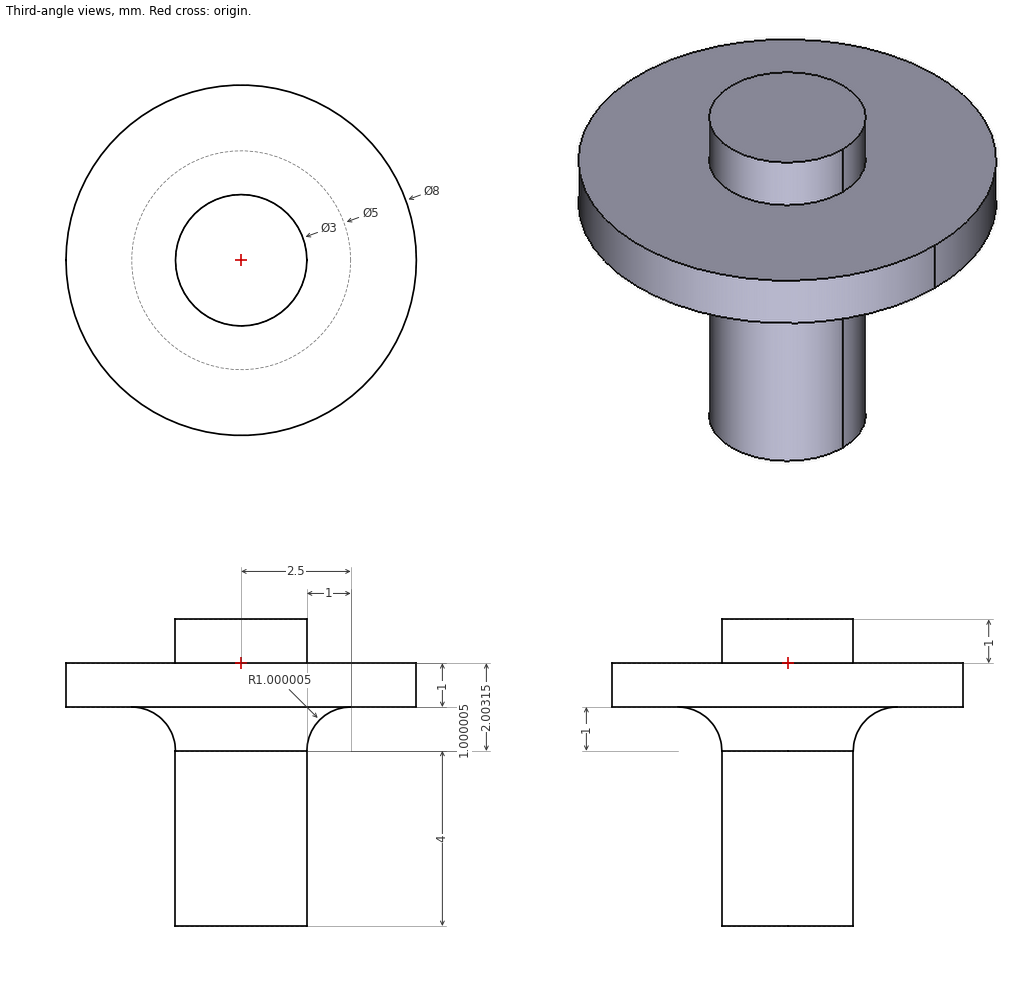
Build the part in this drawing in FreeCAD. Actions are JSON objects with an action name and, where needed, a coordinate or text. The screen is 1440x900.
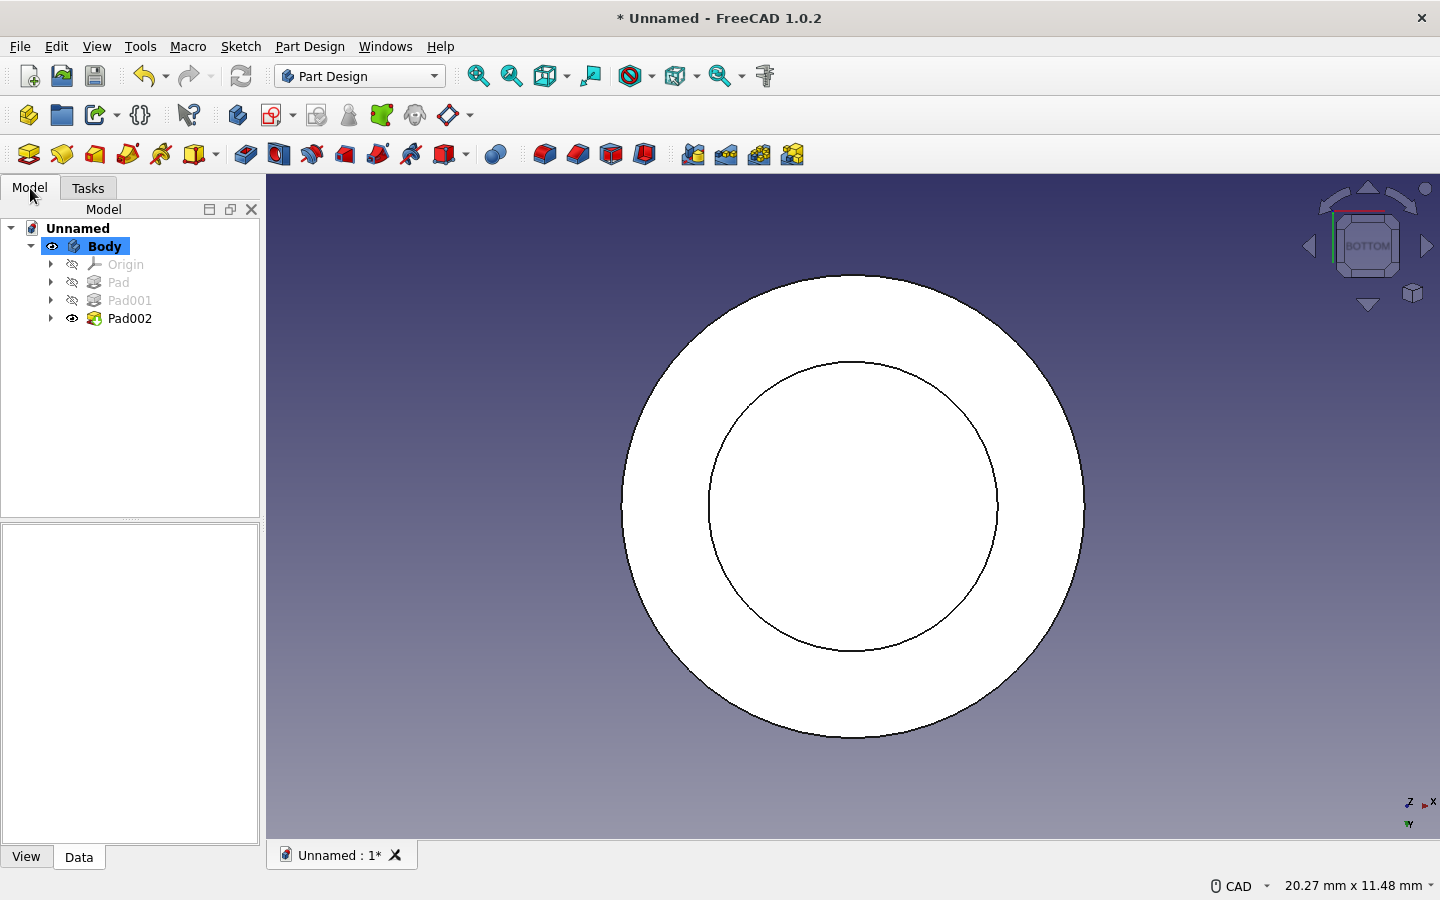
{"action": "left_click", "coordinate": [51, 264]}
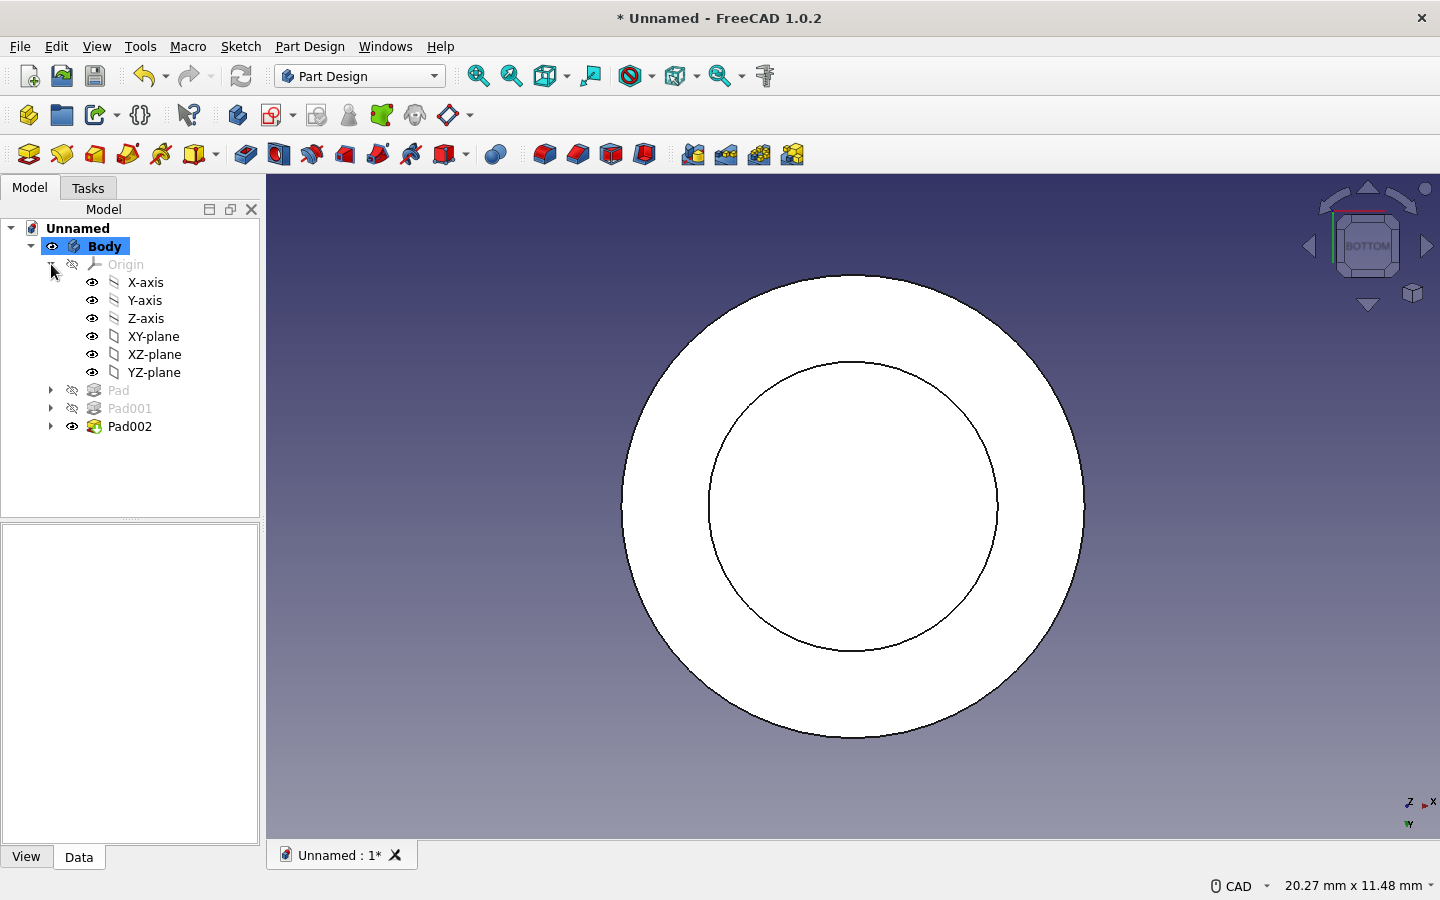
{"action": "left_click", "coordinate": [137, 336]}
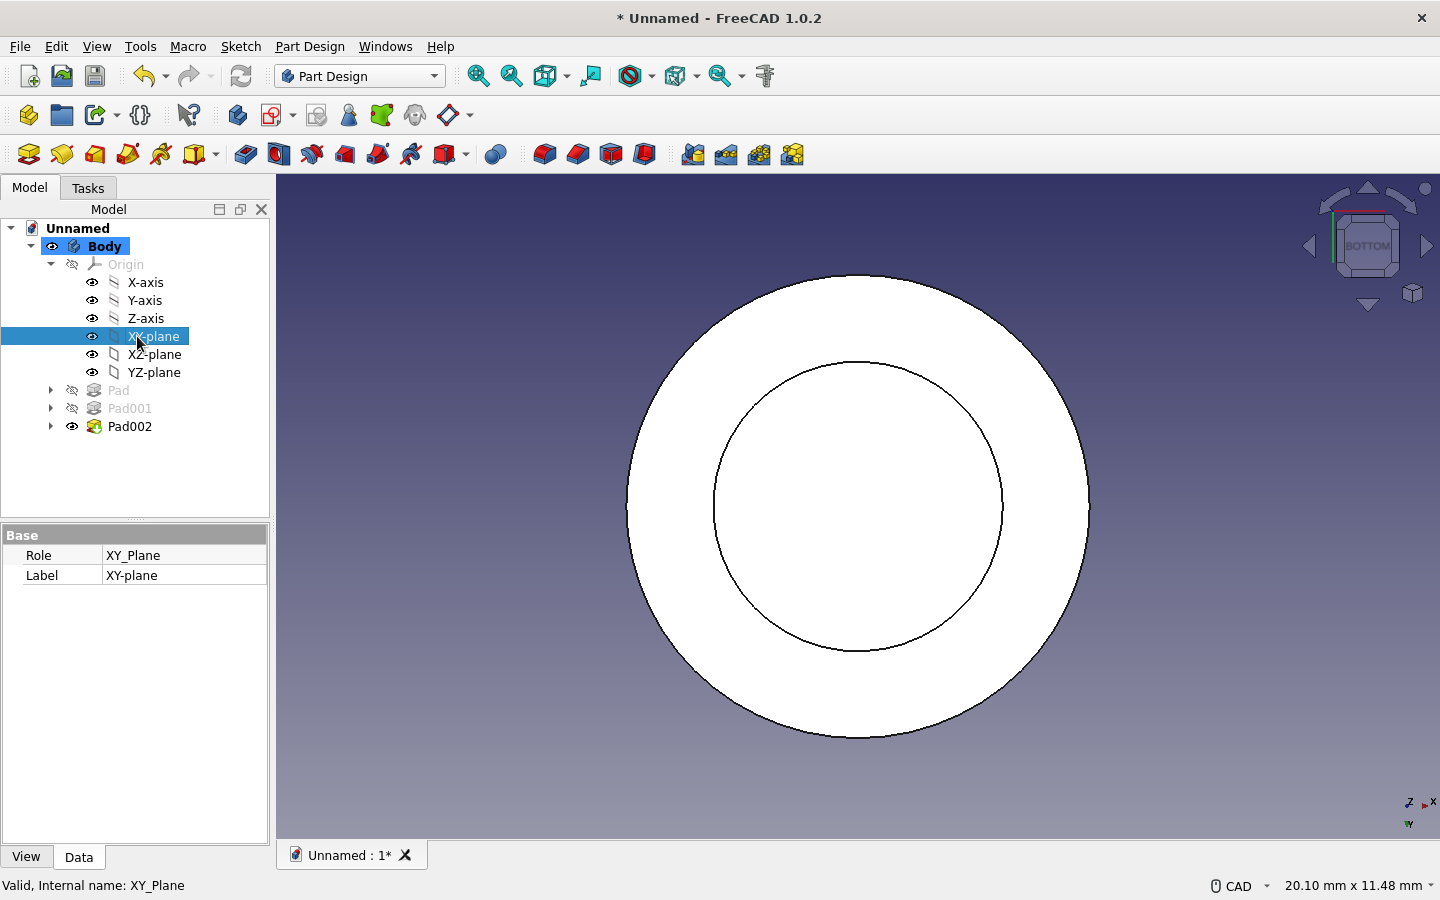
{"action": "left_click", "coordinate": [448, 116]}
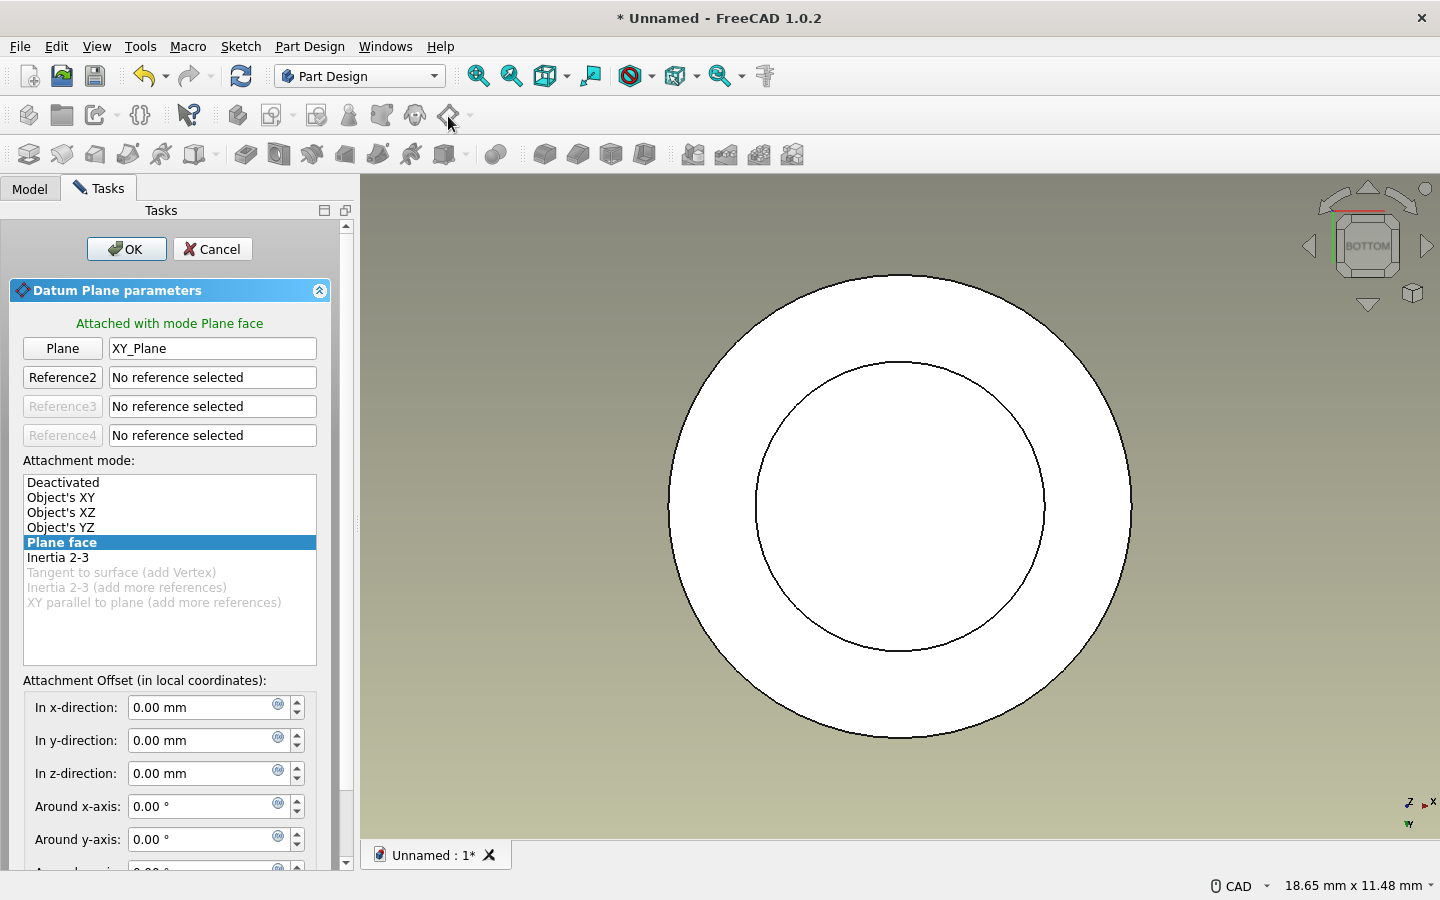
{"action": "triple_click", "coordinate": [210, 774]}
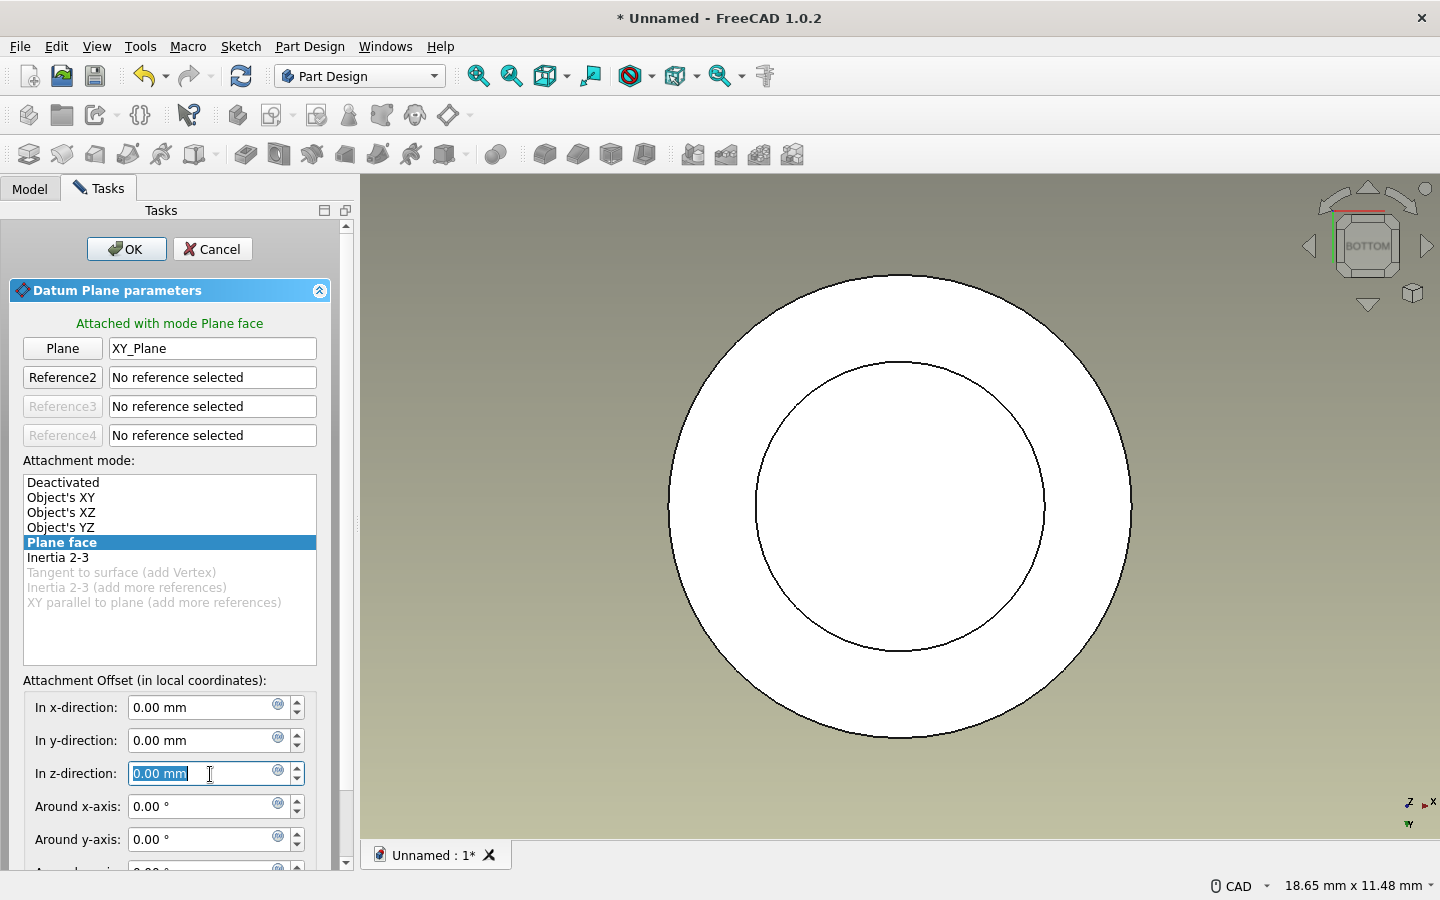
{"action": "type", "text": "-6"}
{"action": "key", "text": "Tab"}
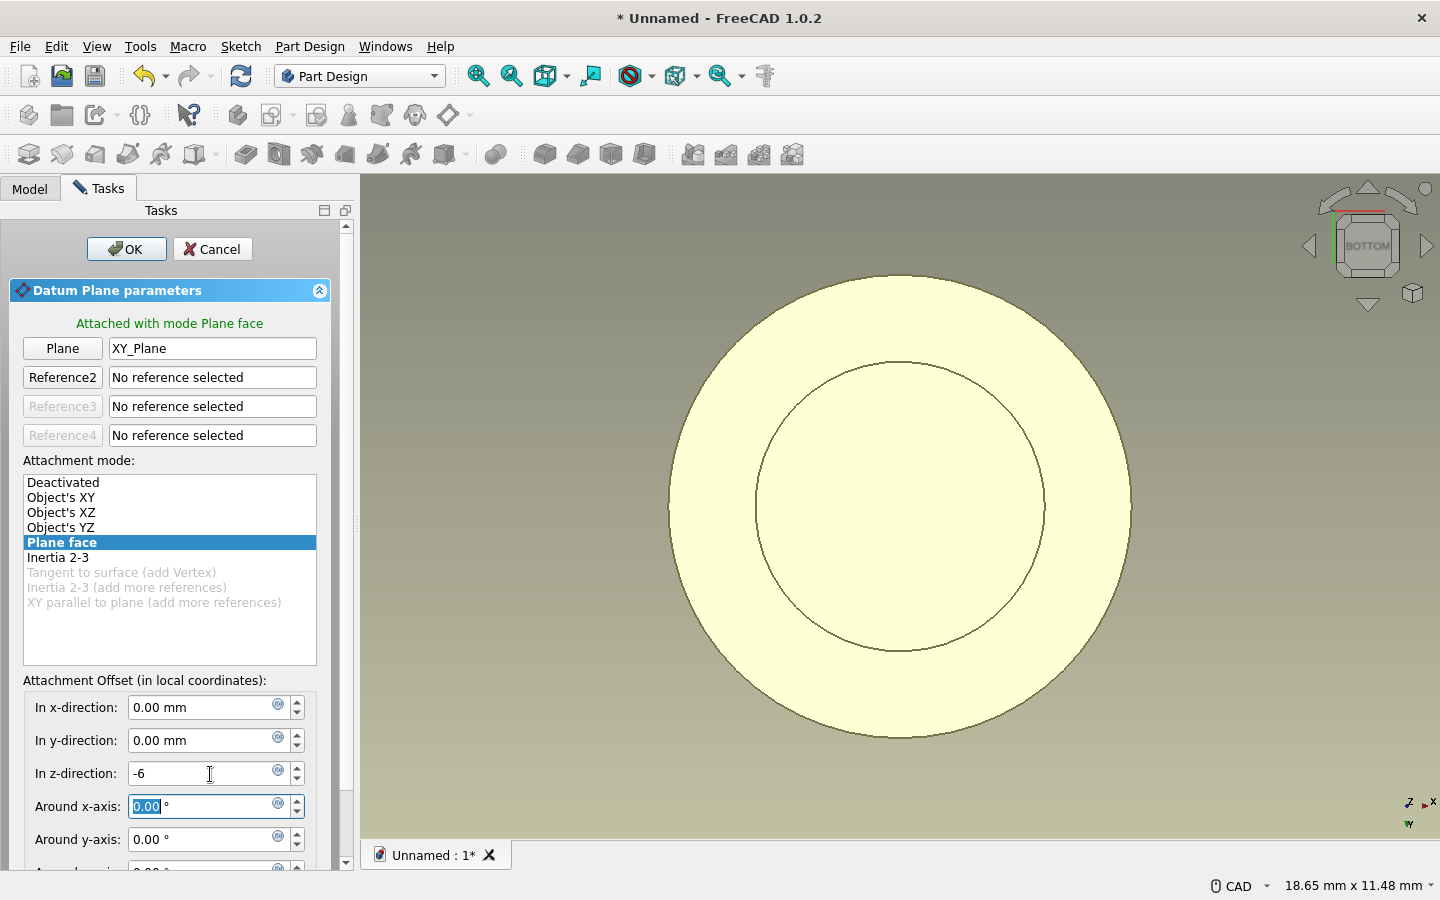
{"action": "left_click", "coordinate": [127, 249]}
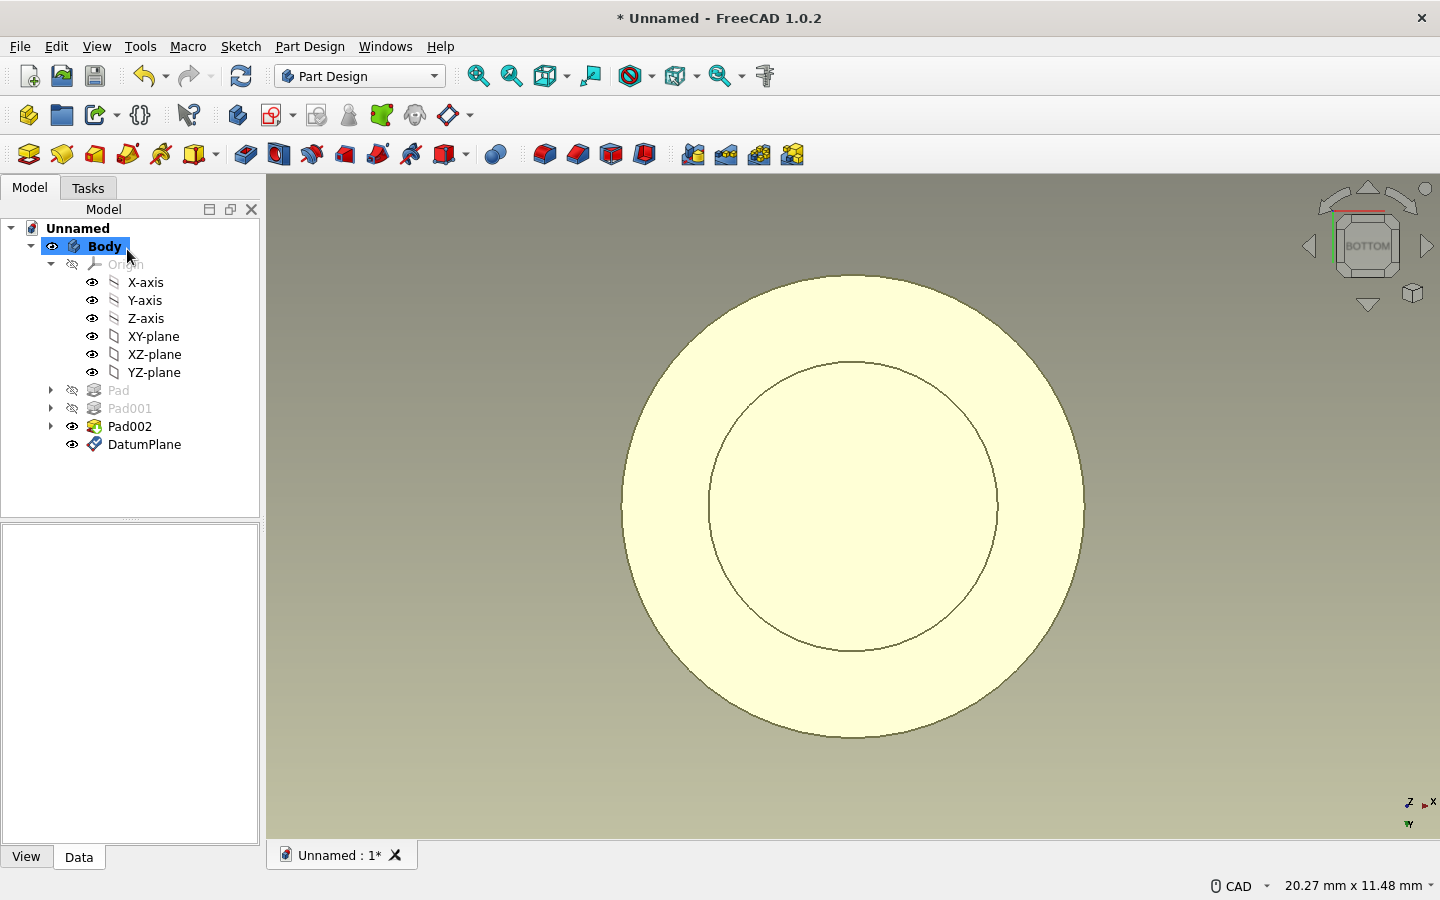
{"action": "left_click", "coordinate": [117, 444]}